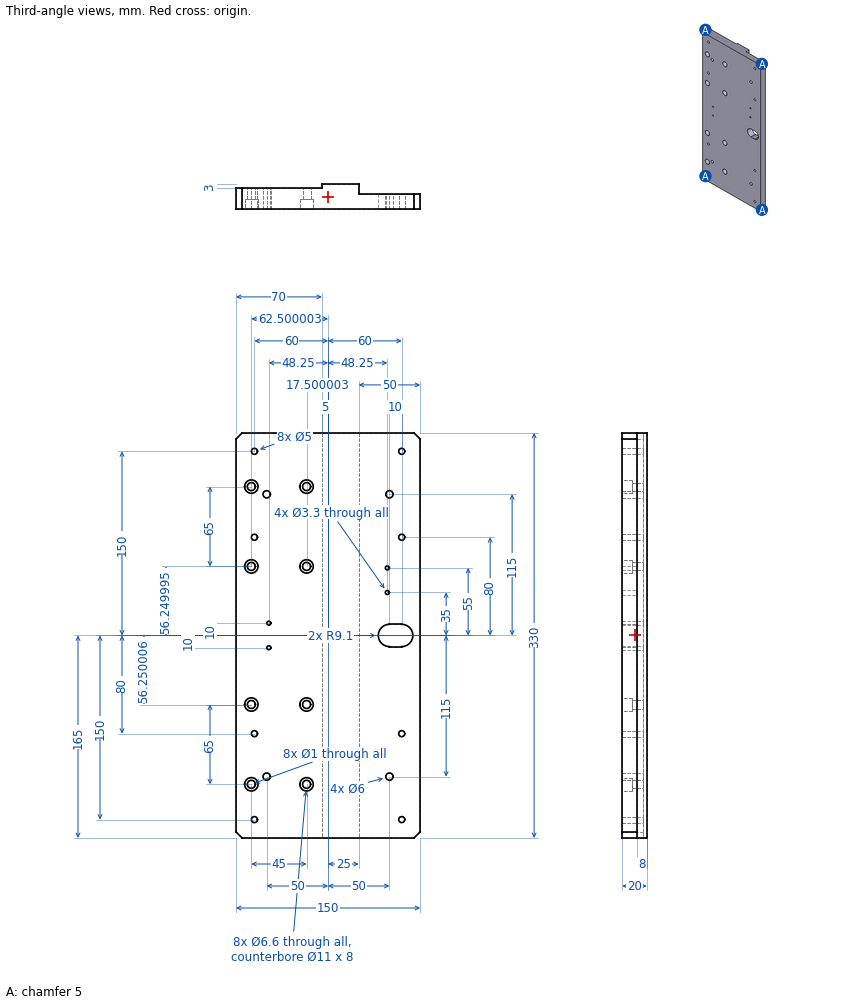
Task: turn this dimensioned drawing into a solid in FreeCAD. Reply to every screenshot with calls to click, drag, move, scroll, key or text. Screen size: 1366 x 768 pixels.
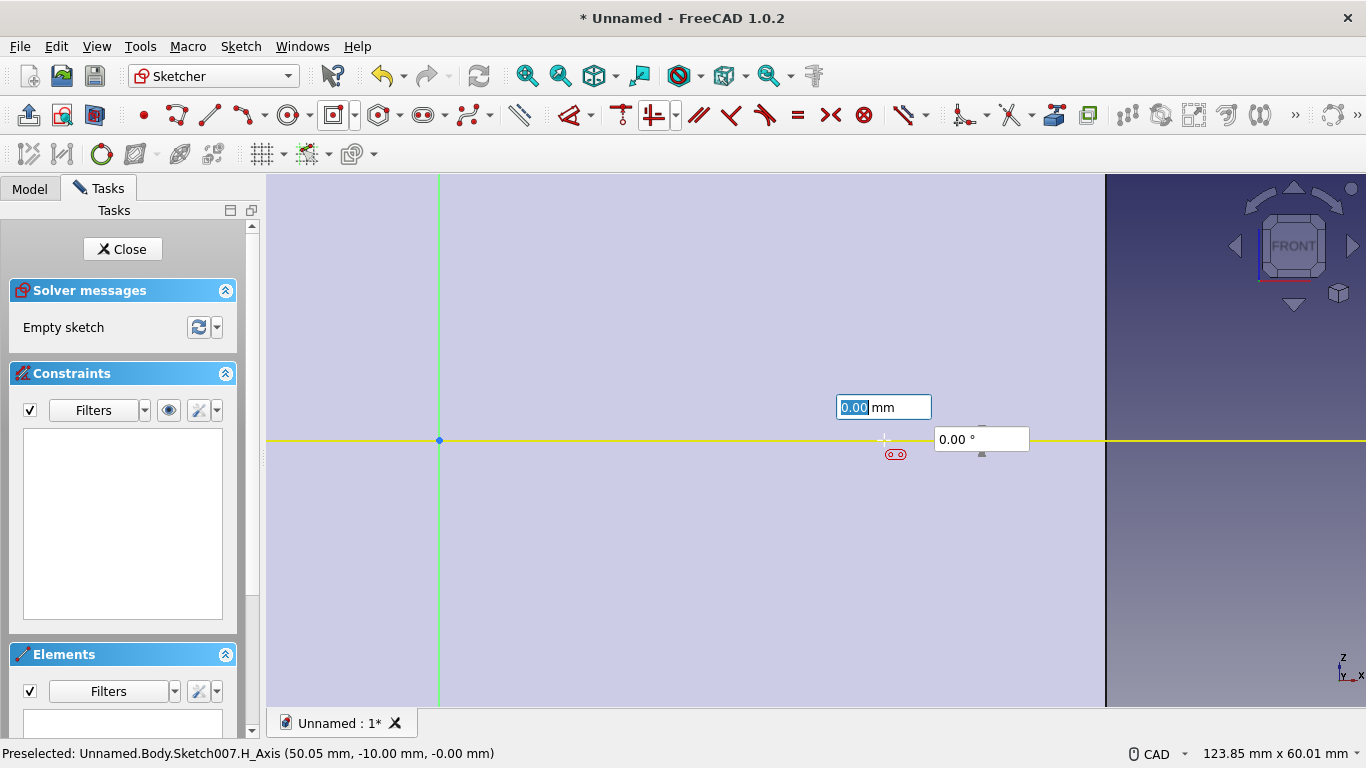
click(972, 431)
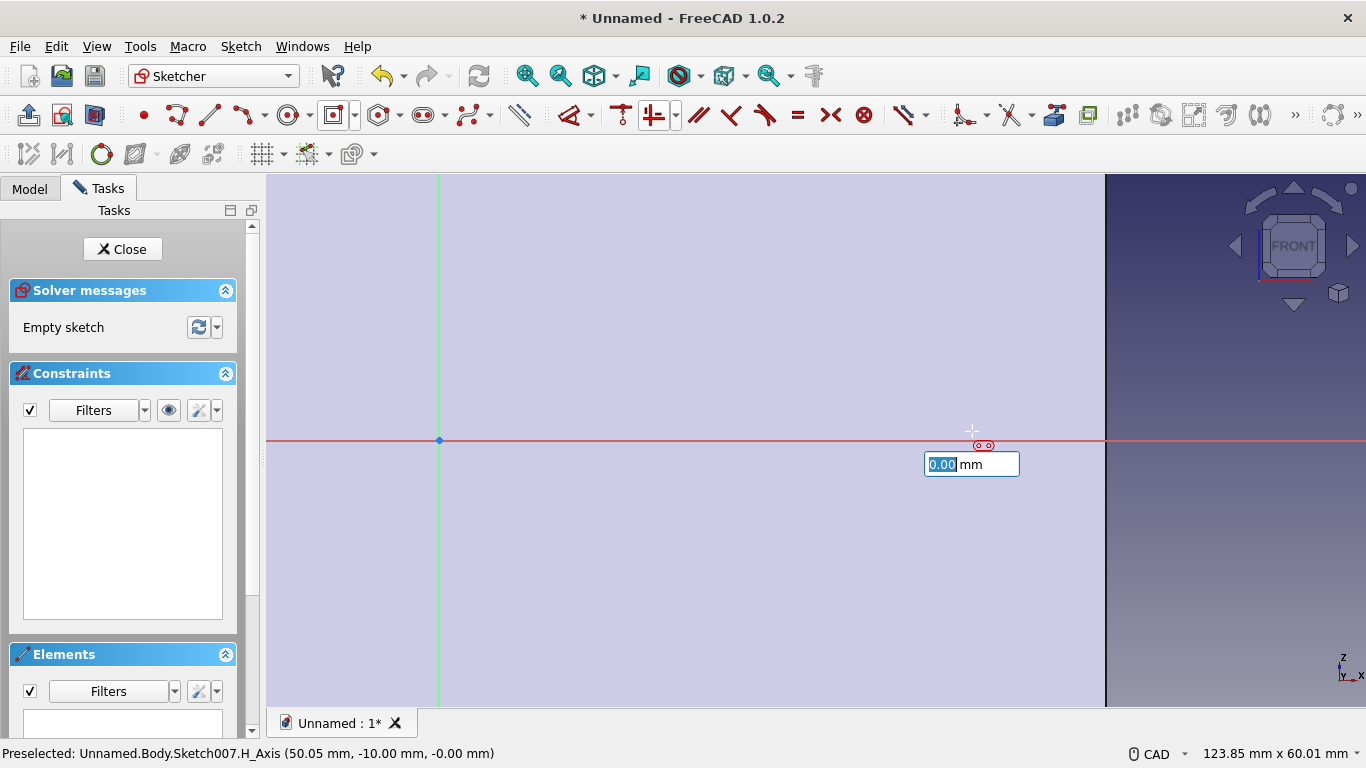
click(928, 360)
key(Escape)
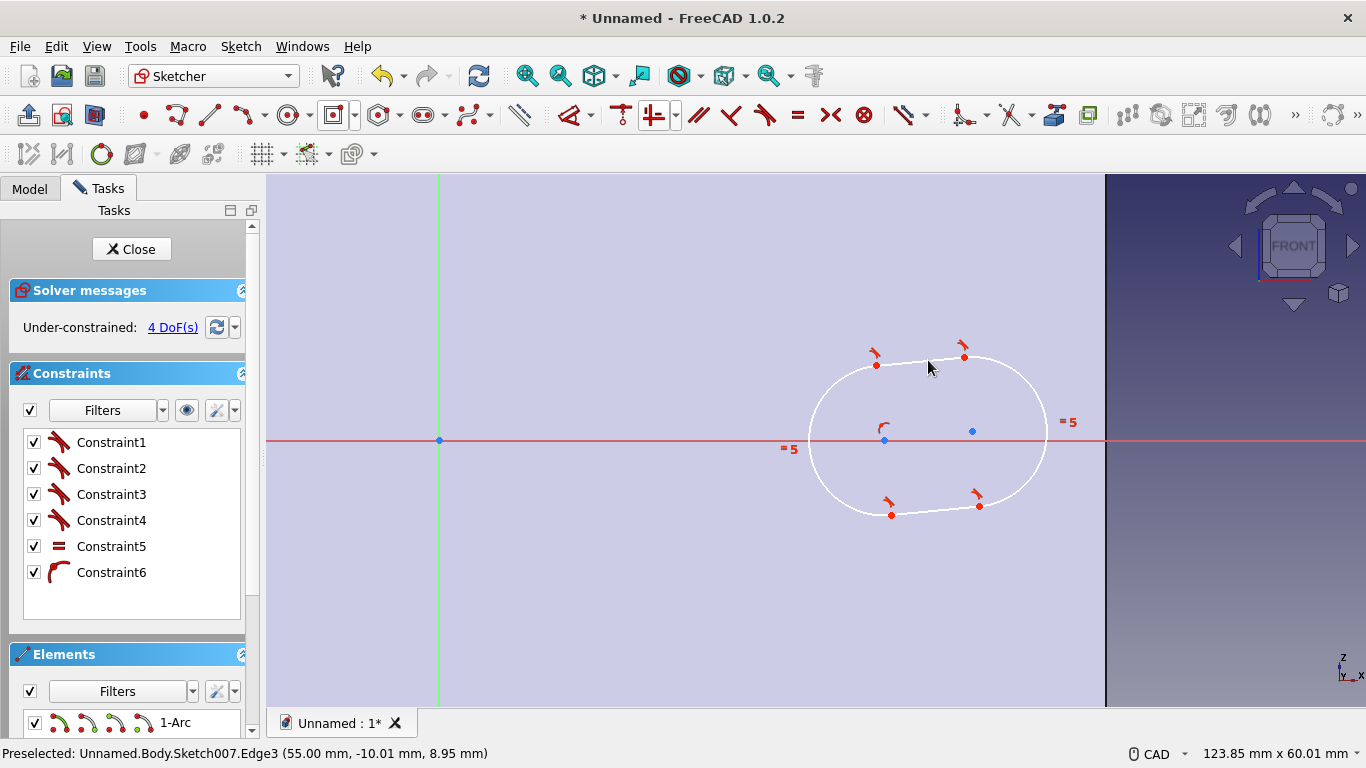
click(903, 363)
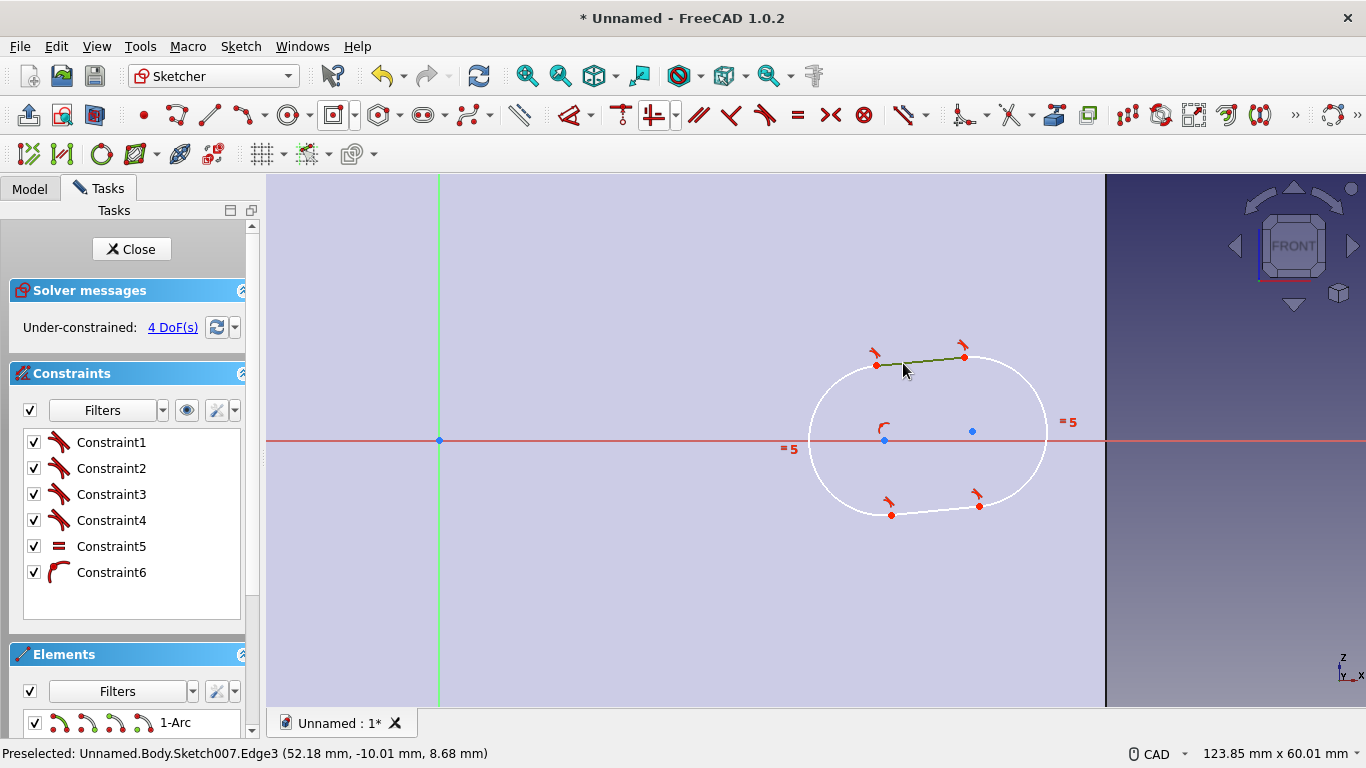
key(h)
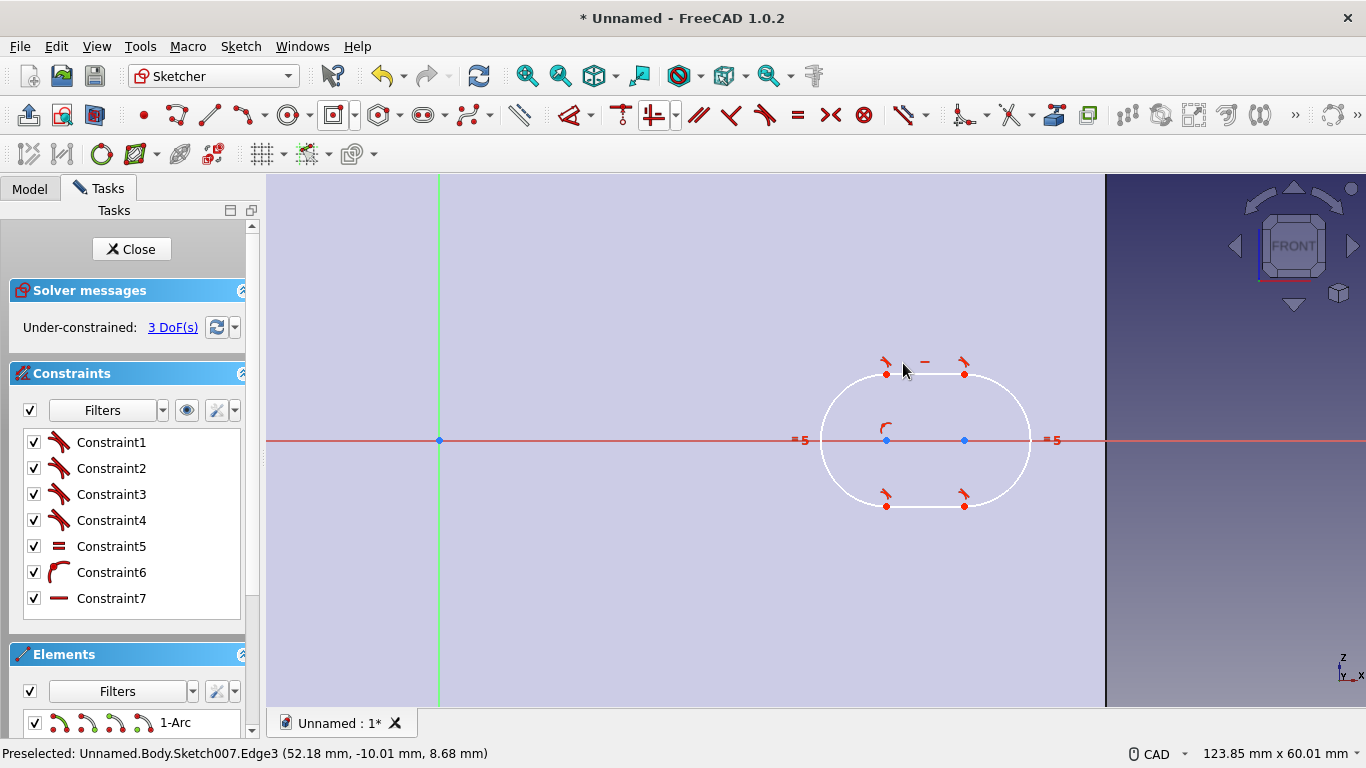
click(568, 116)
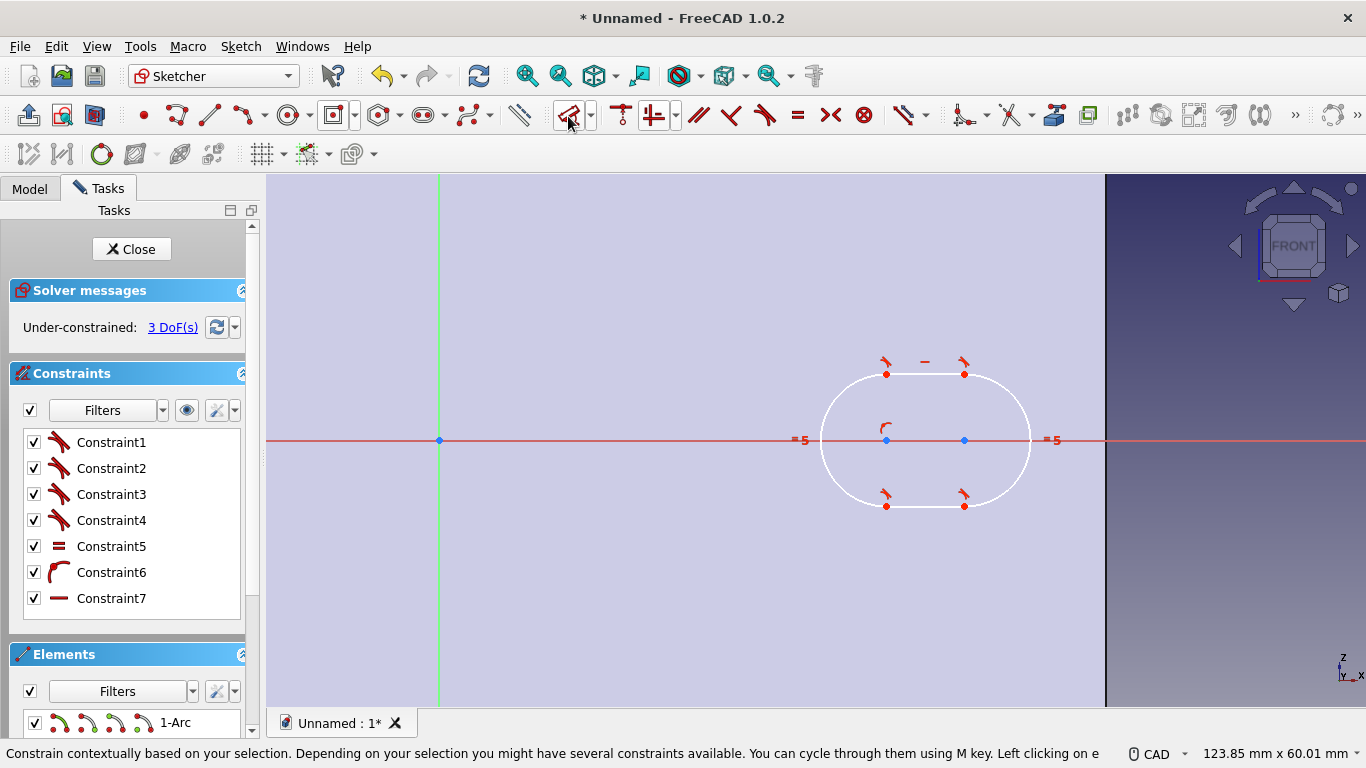
click(833, 402)
click(807, 383)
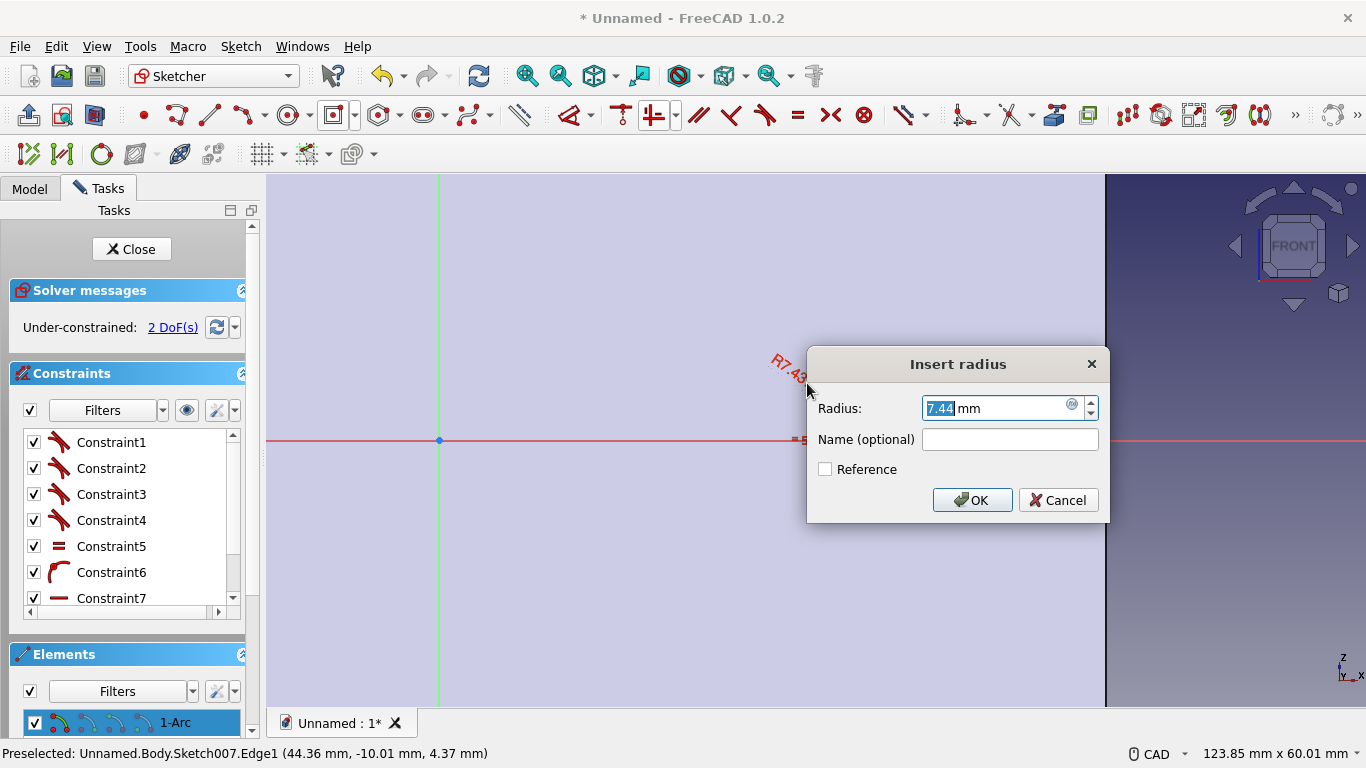
text(9.1)
key(Return)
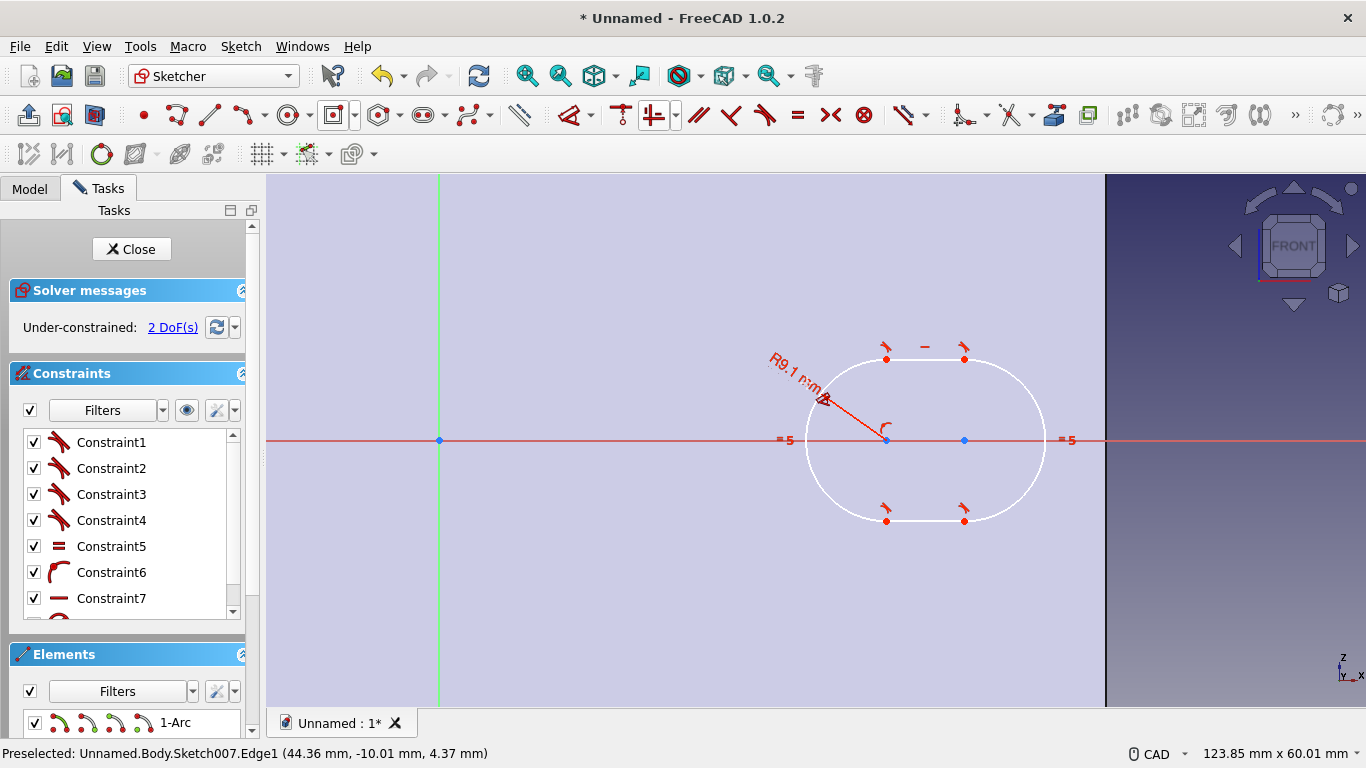
click(910, 360)
click(926, 326)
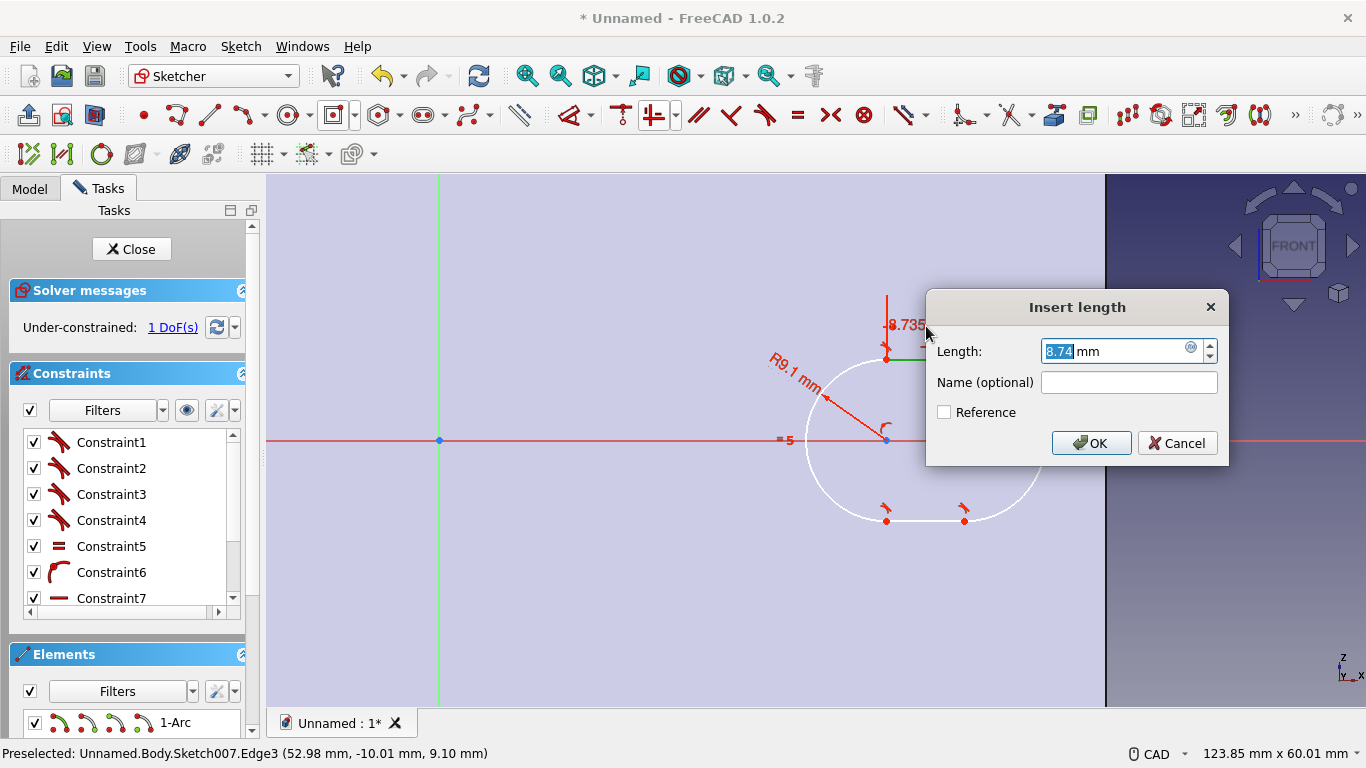
text(10)
key(Return)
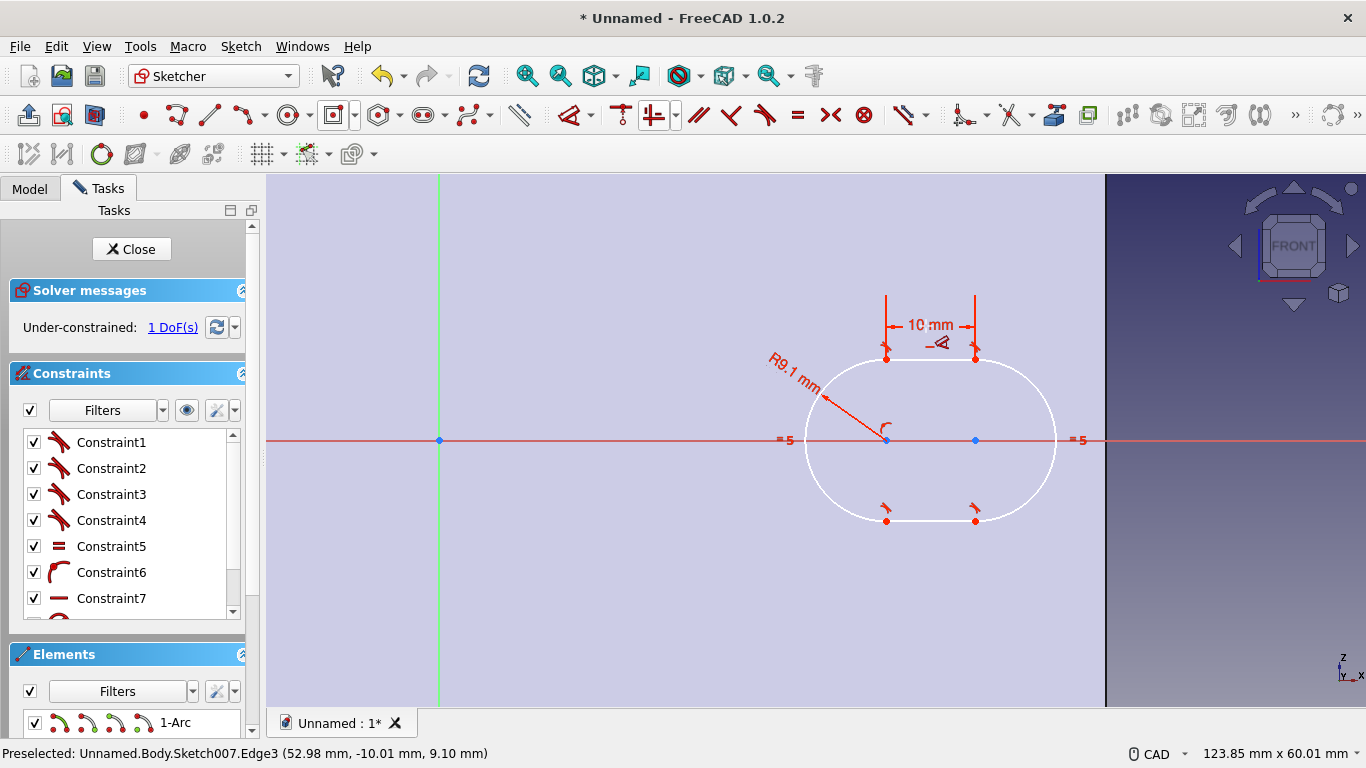
click(886, 360)
click(663, 326)